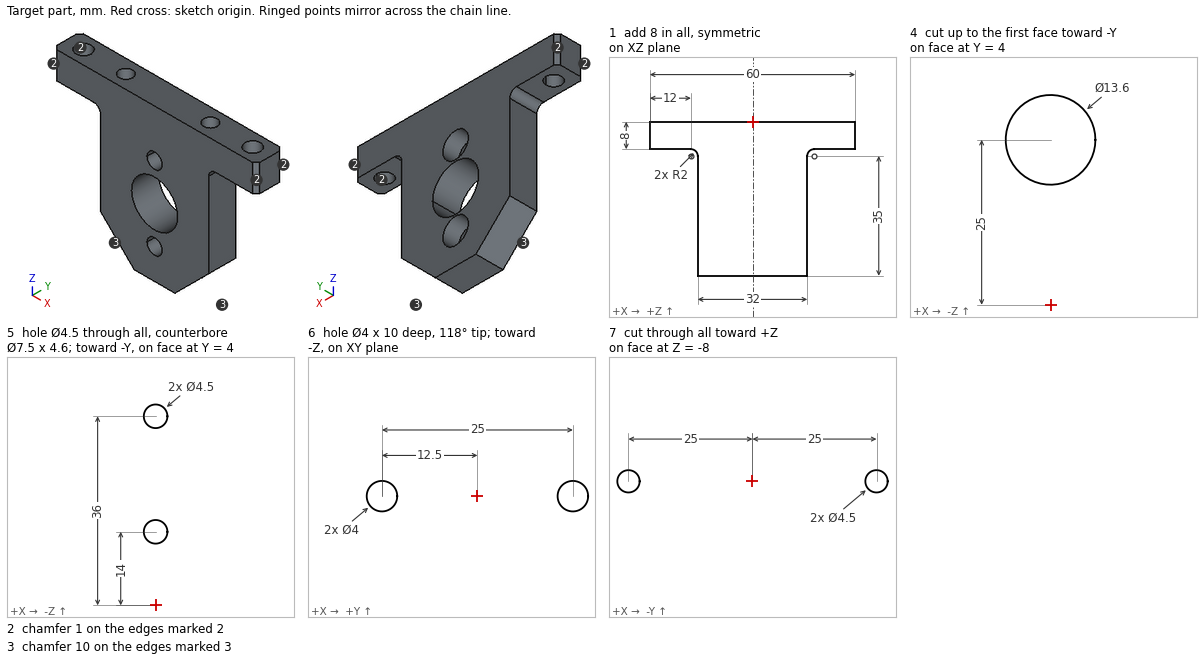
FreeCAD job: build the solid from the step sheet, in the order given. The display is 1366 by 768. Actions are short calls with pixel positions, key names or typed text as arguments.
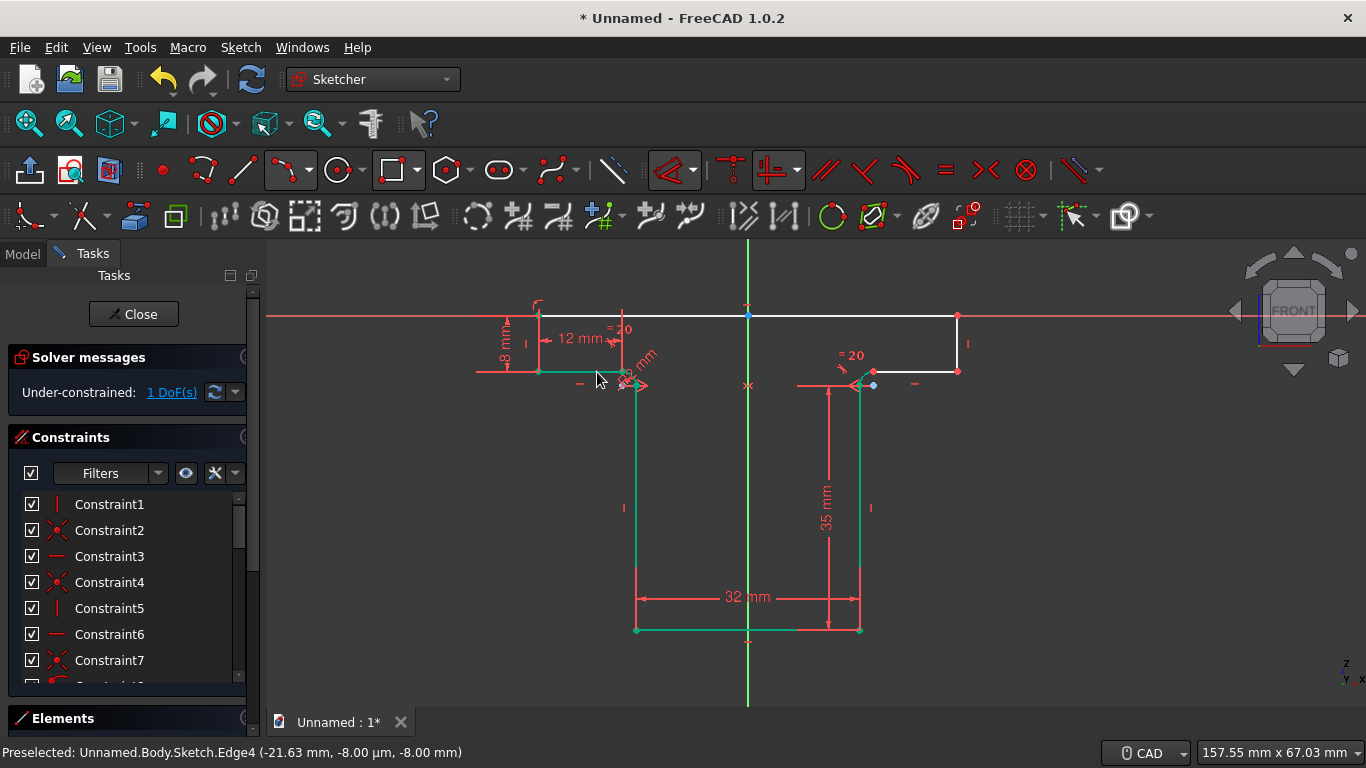
click(664, 316)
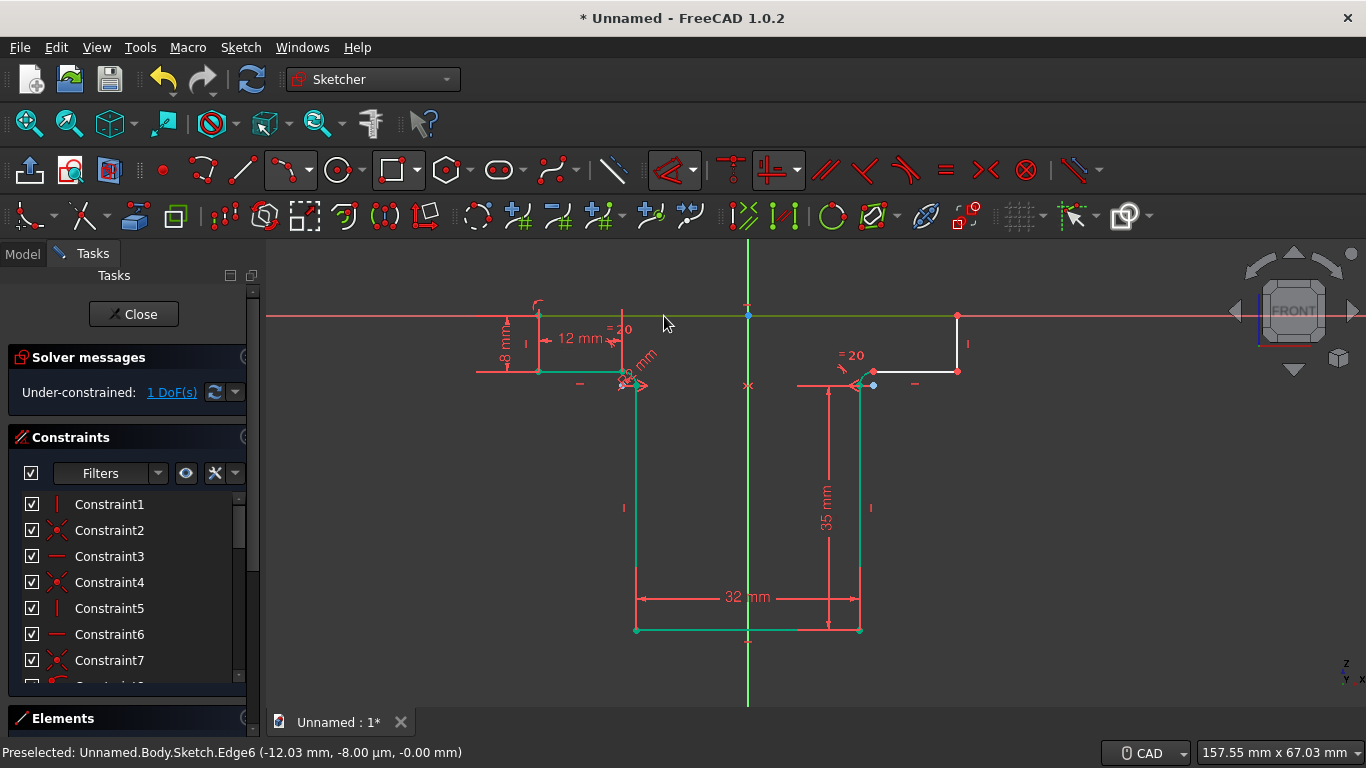
key(l)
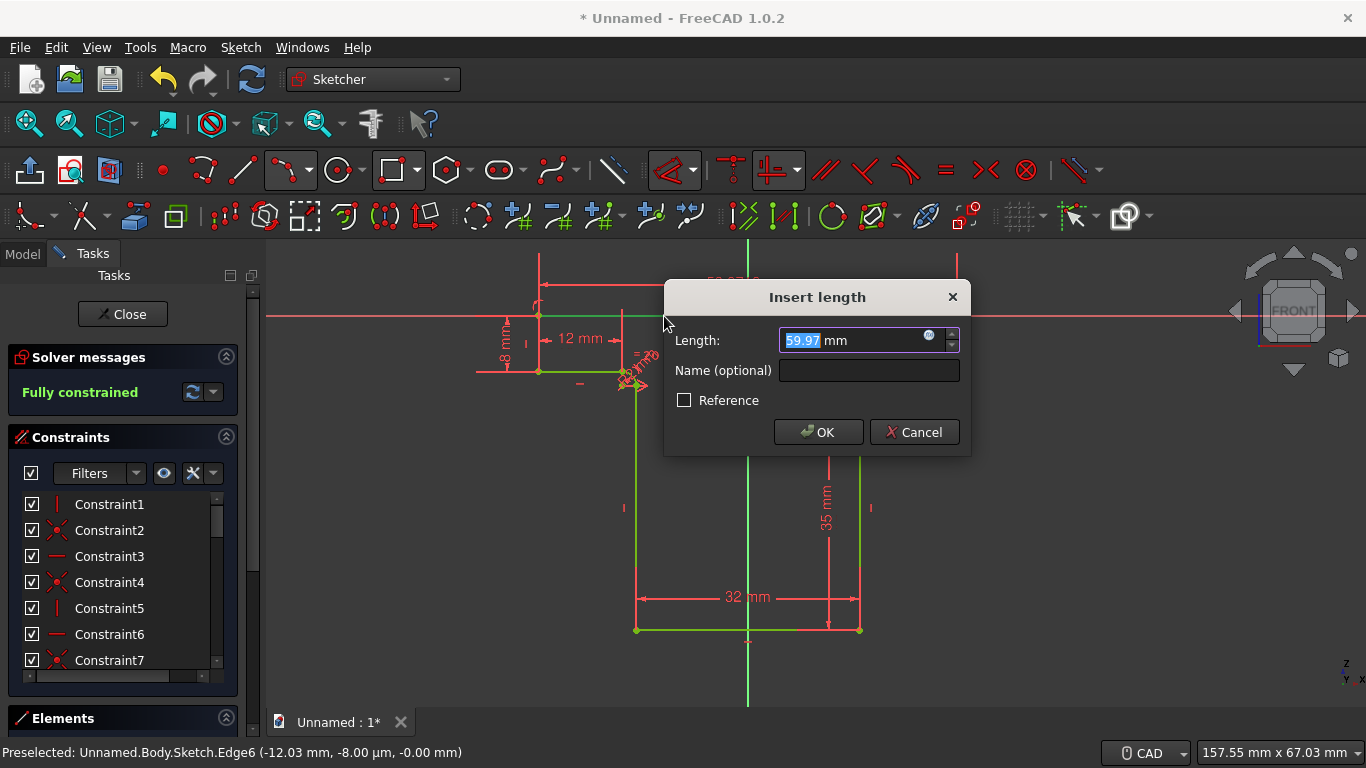
text(60)
key(Return)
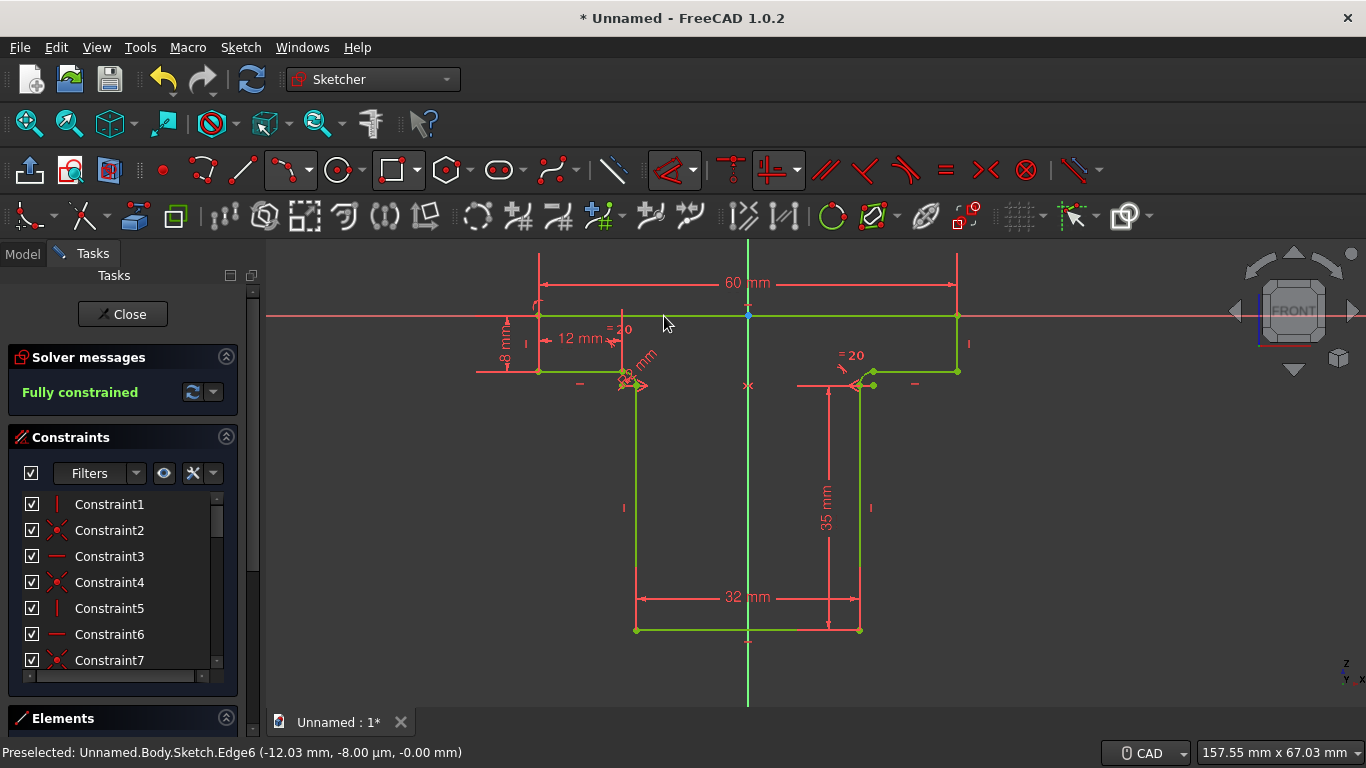
click(123, 314)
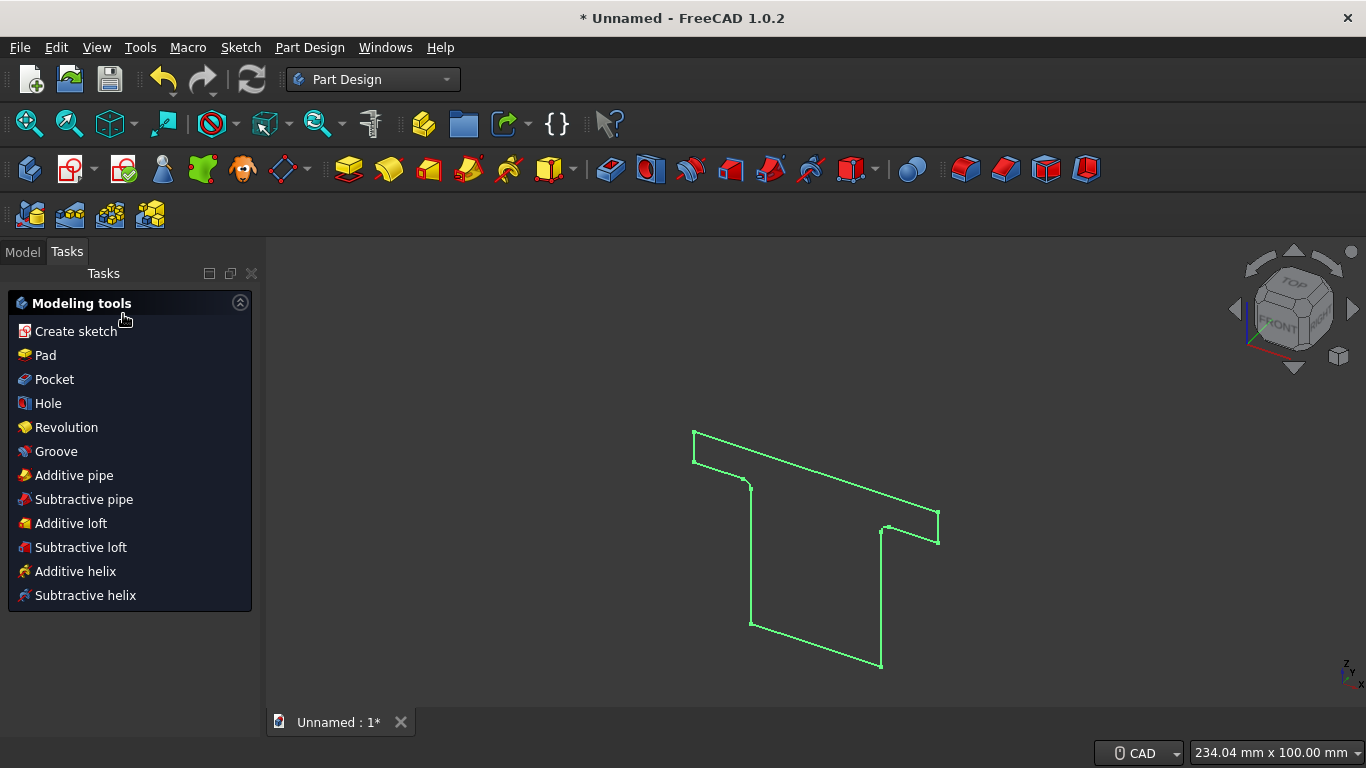
click(350, 170)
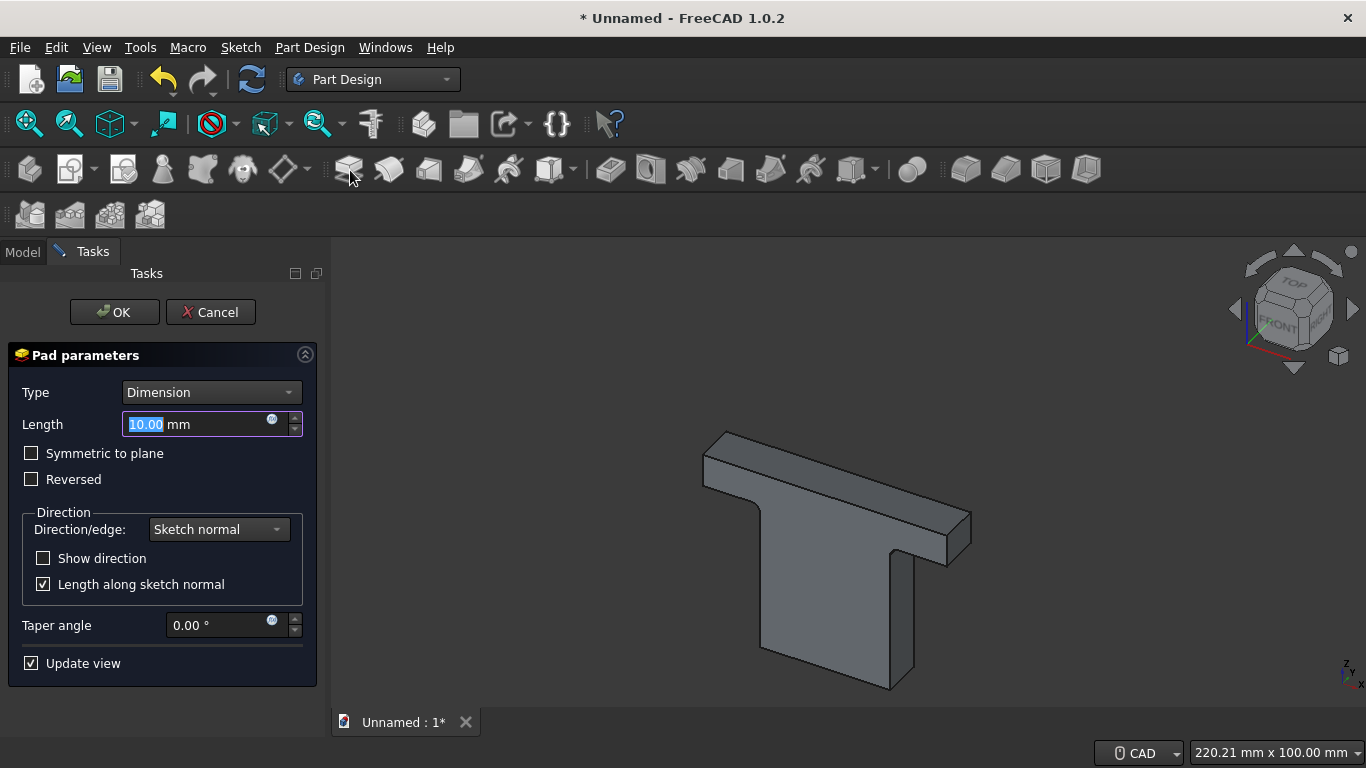
text(8)
key(Tab)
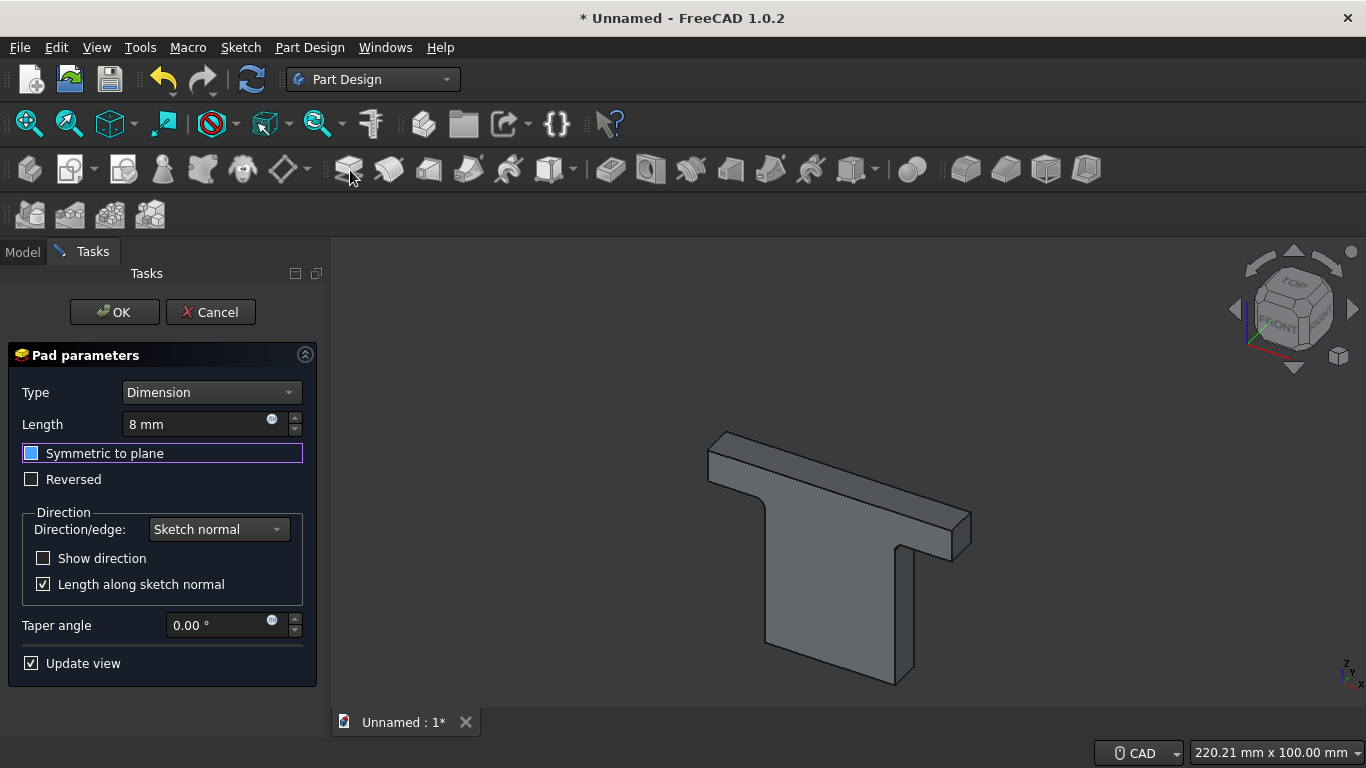
click(30, 453)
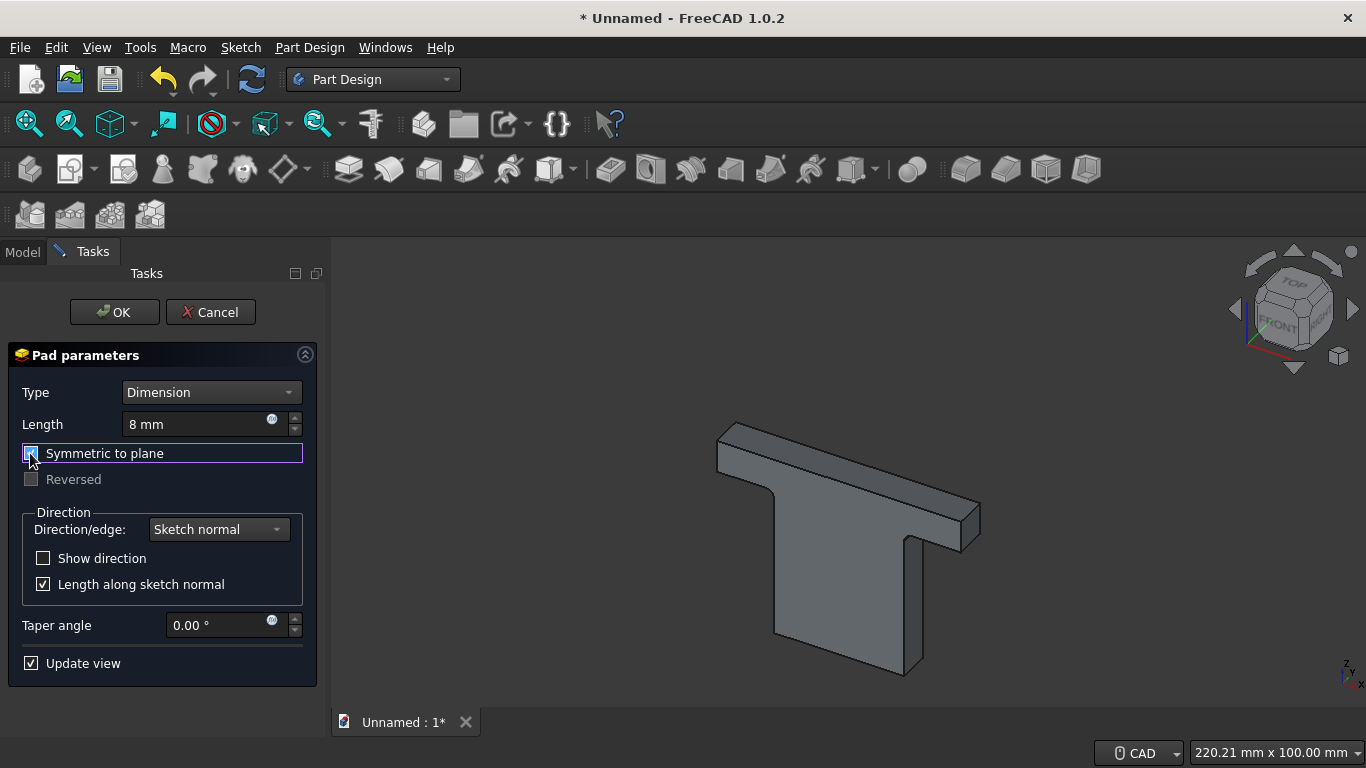
click(115, 312)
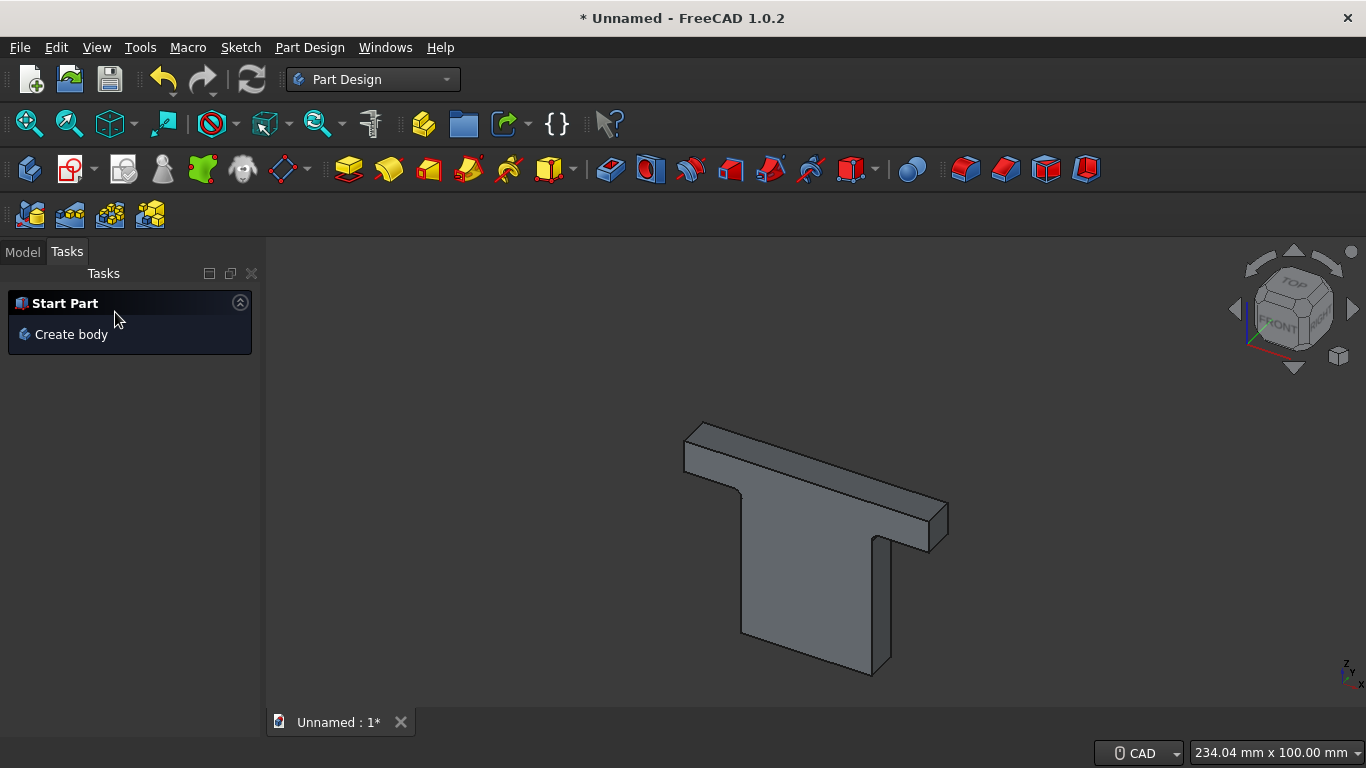
click(929, 536)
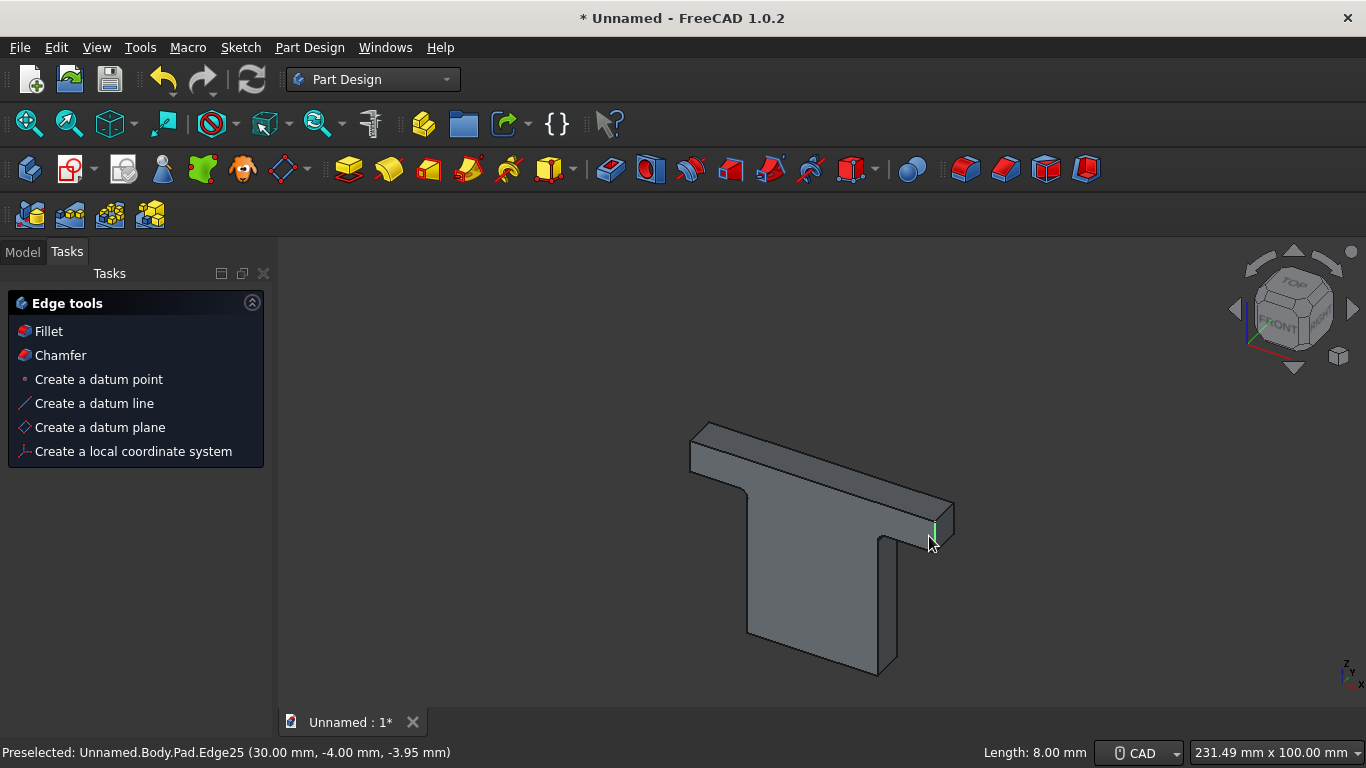
key(0)